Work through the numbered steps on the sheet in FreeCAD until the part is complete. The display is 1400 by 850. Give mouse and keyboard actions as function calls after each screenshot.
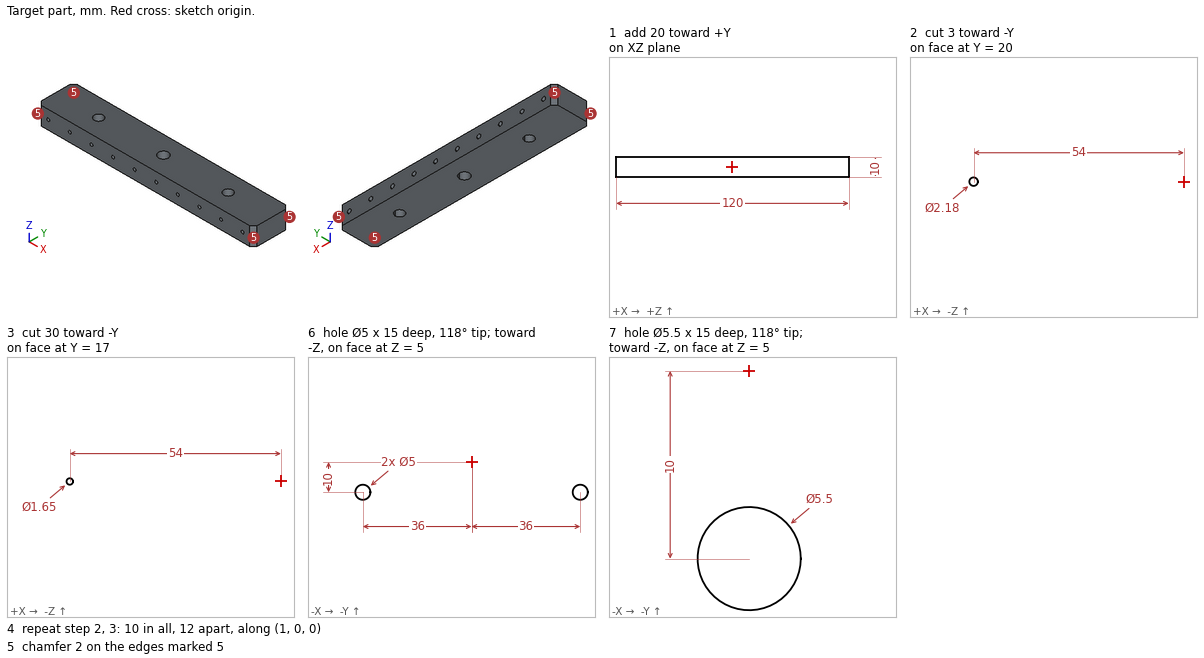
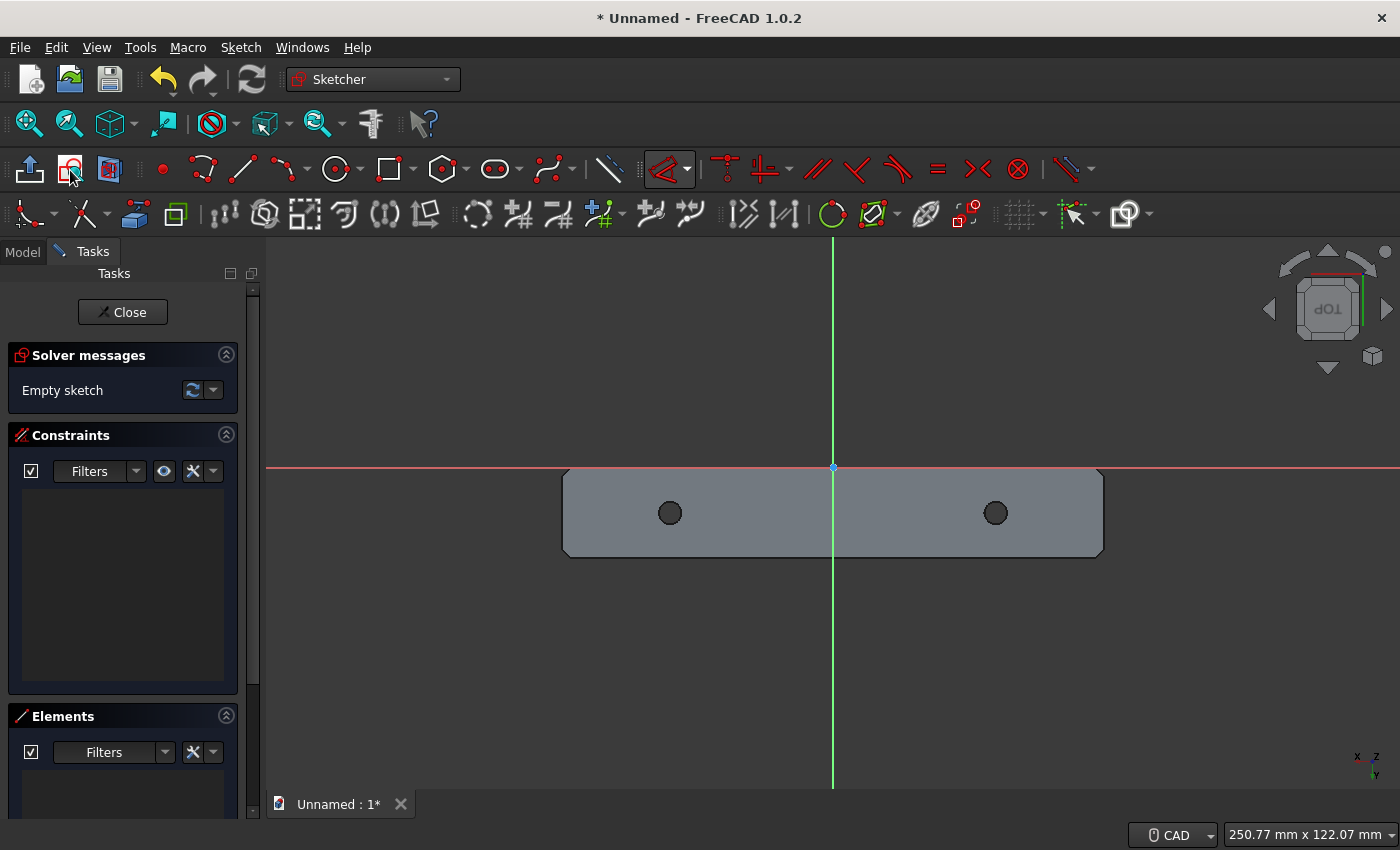
scroll(847, 493, up, 9)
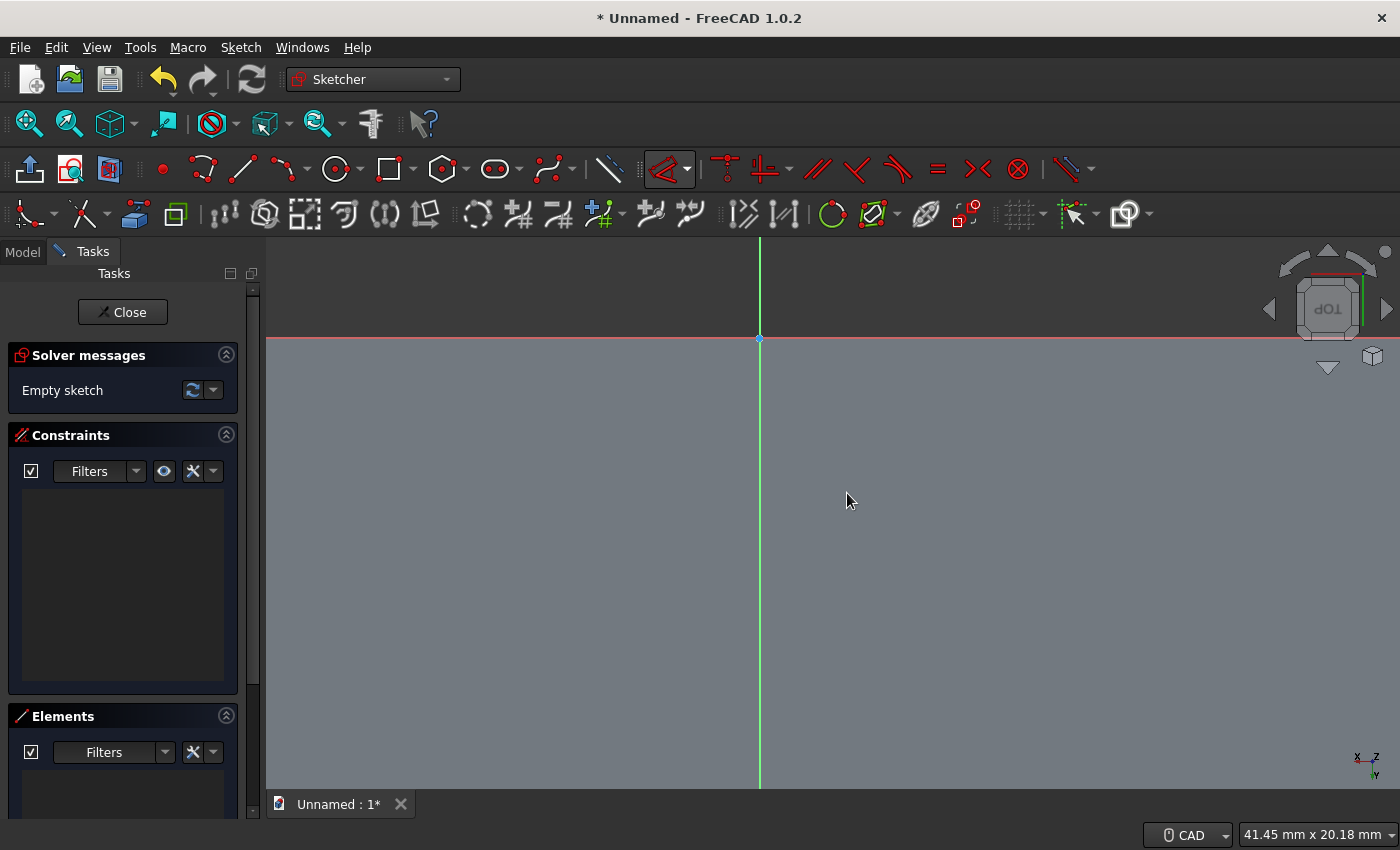
click(336, 170)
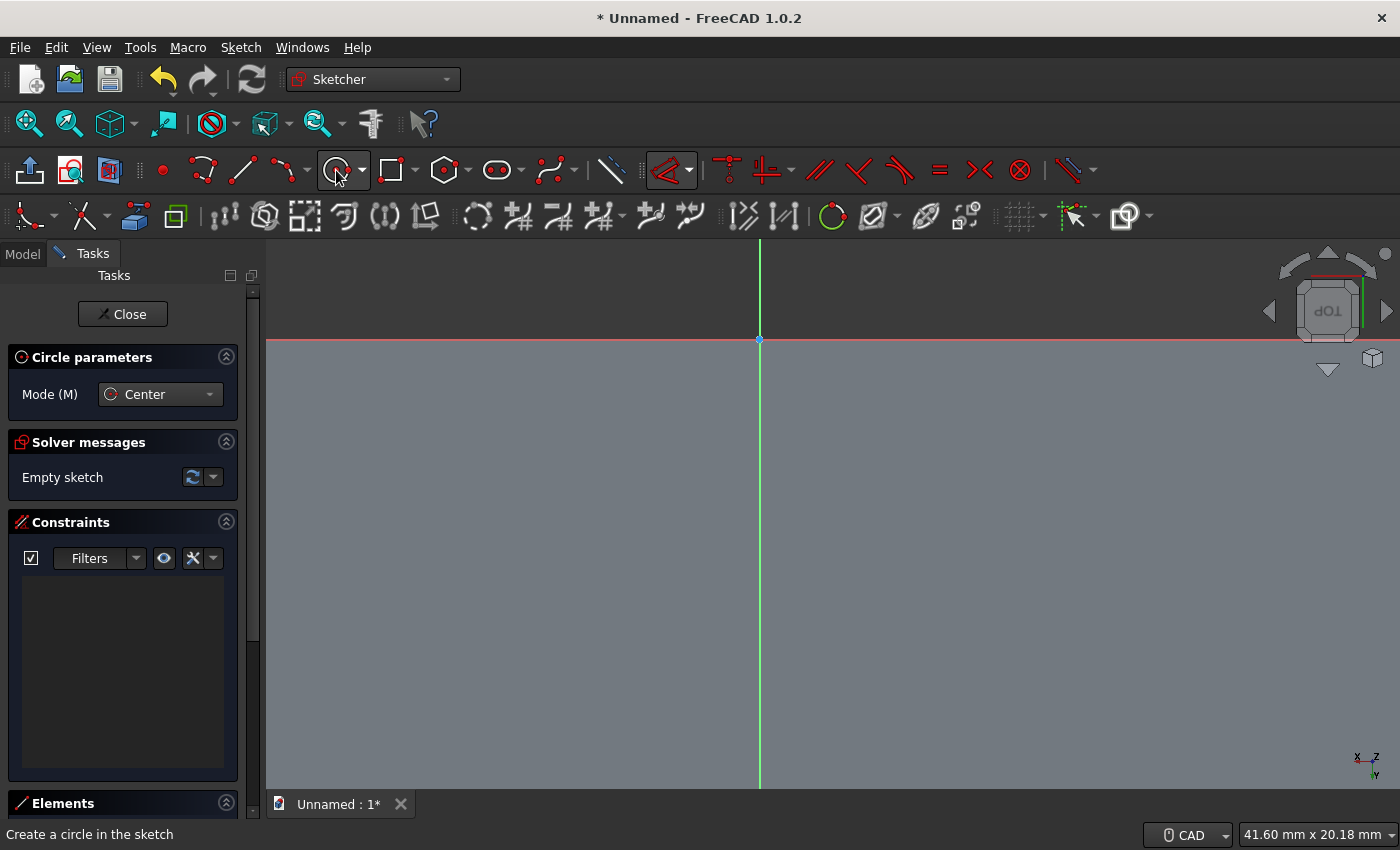
click(760, 612)
click(813, 559)
key(Escape)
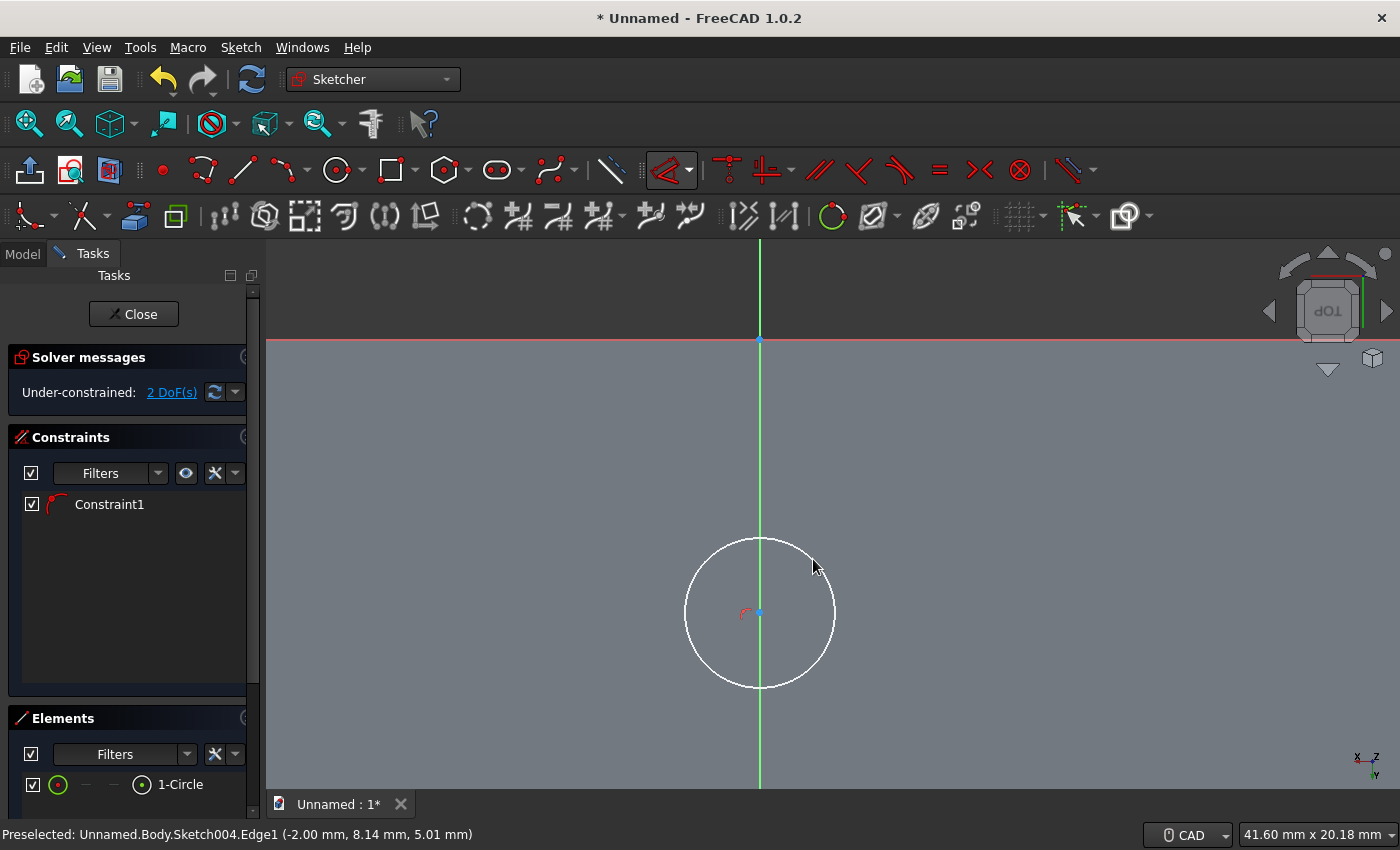
click(813, 560)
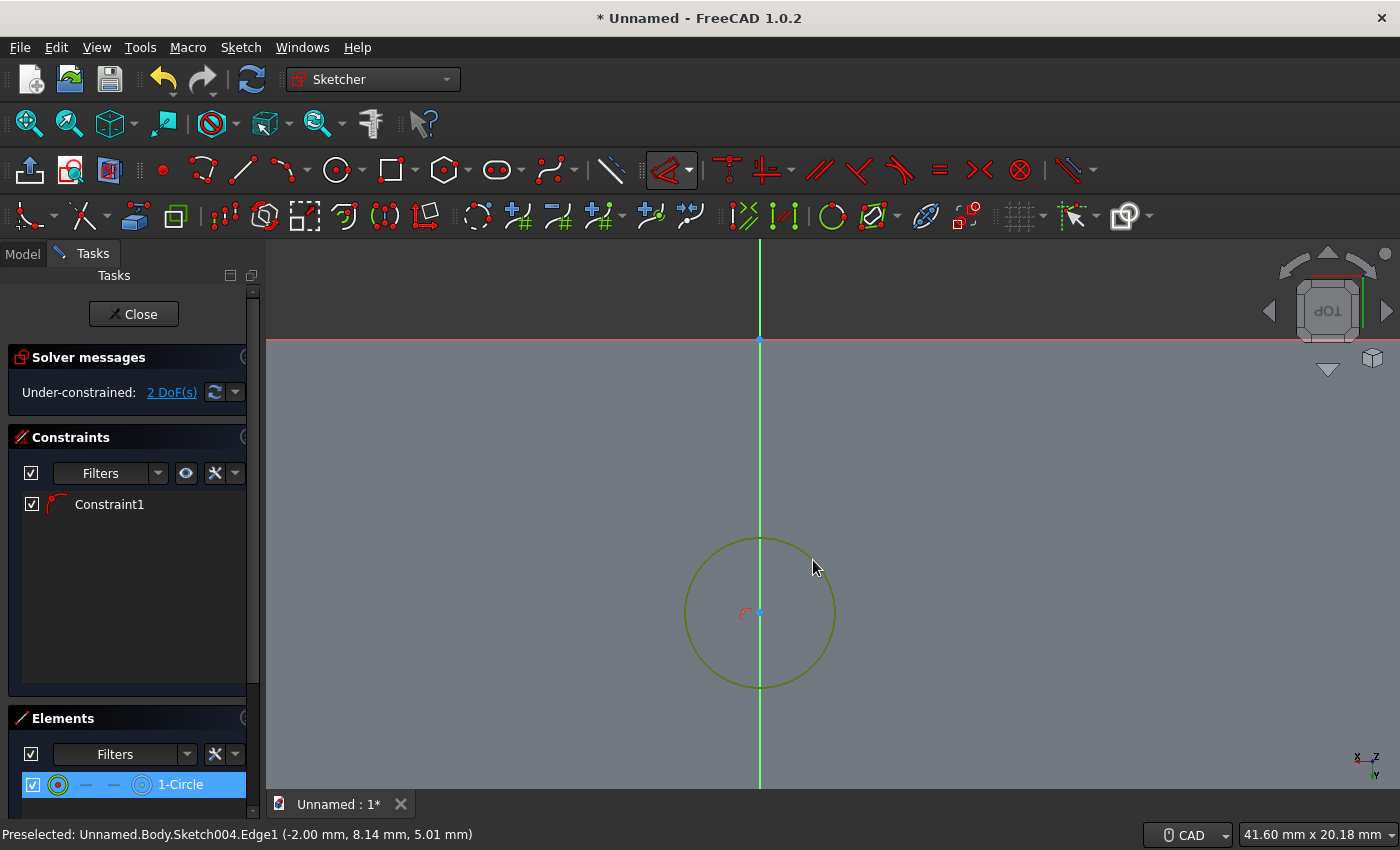
key(k)
key(o)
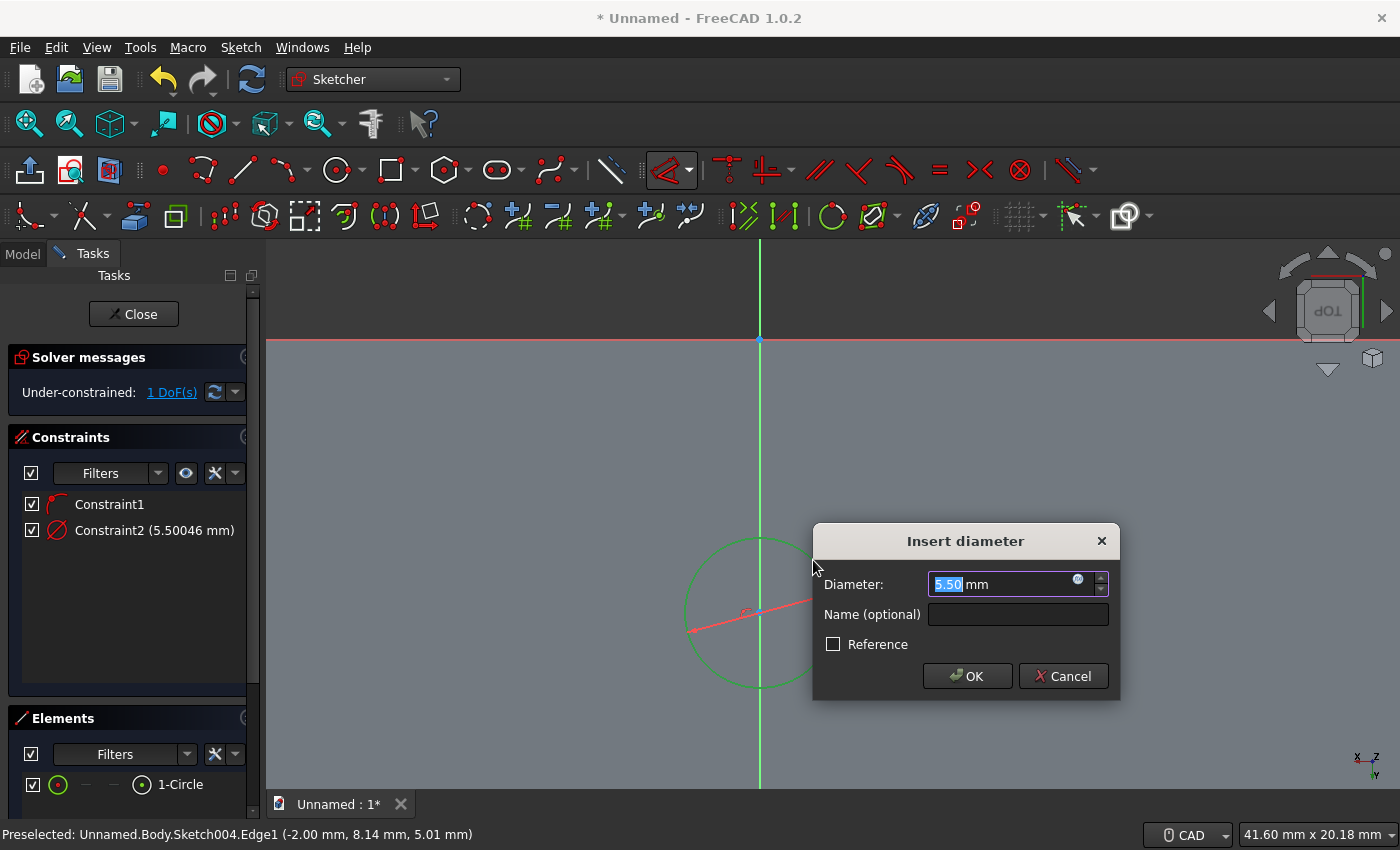
text(5.5)
key(Return)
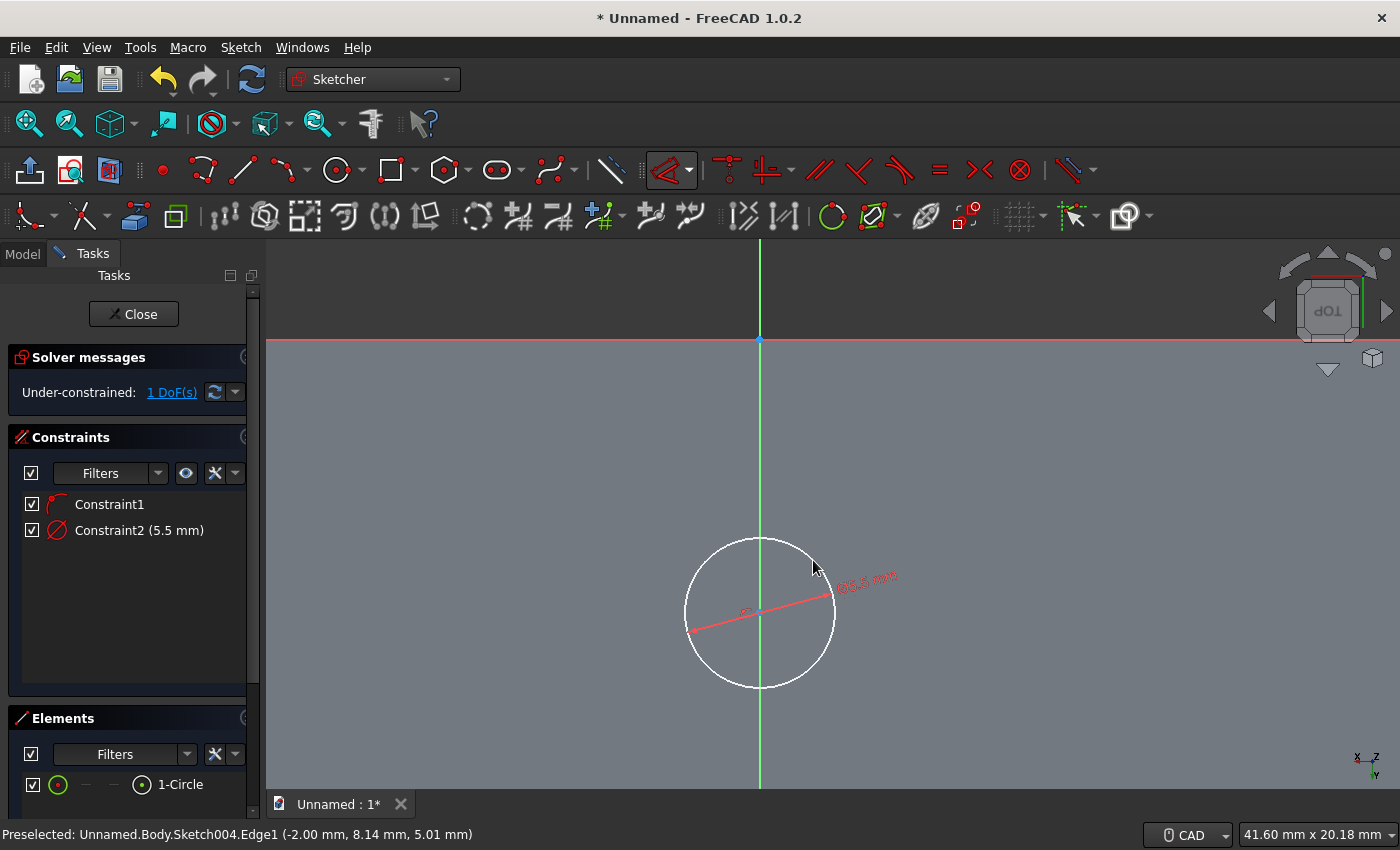
click(760, 613)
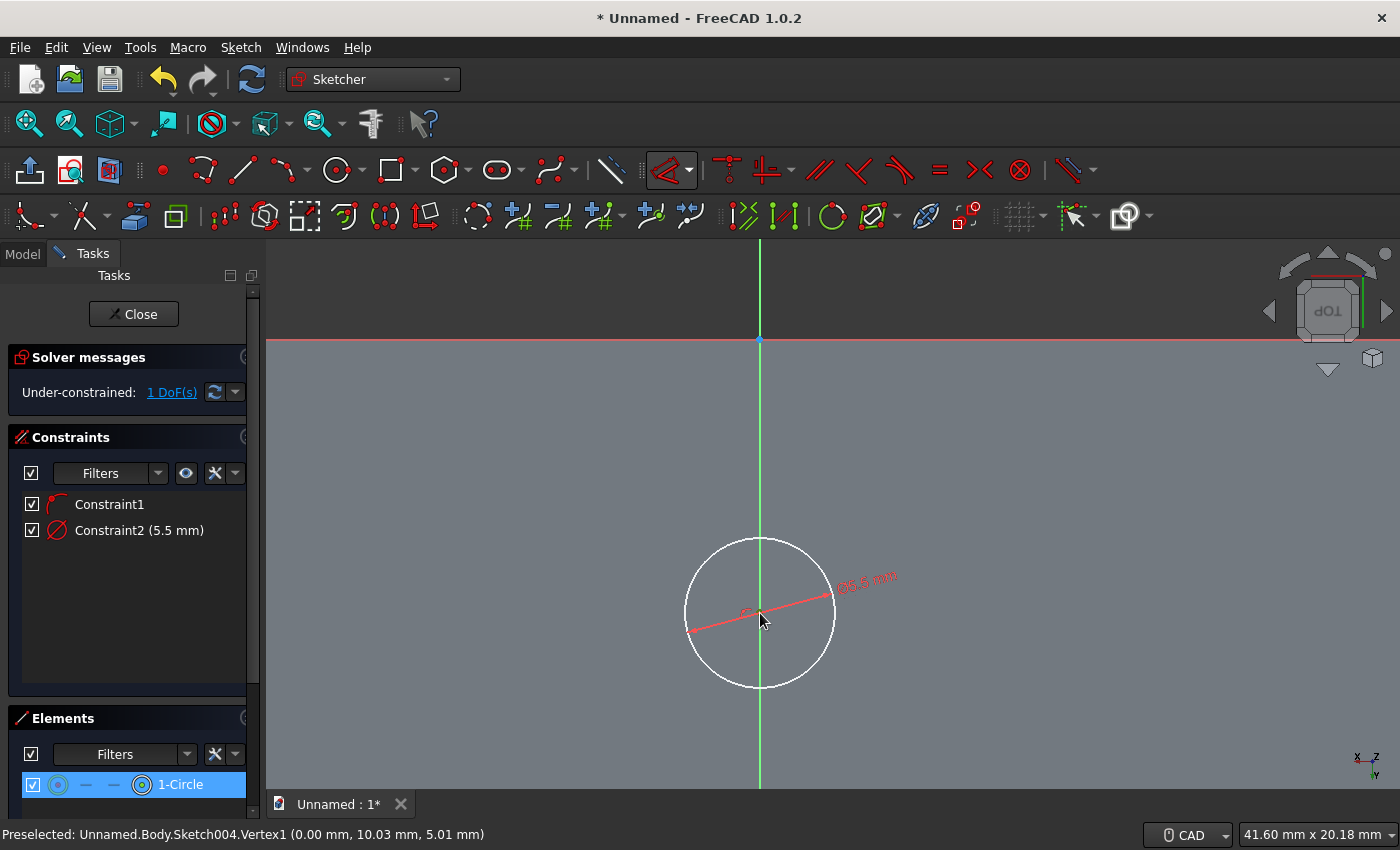
click(692, 170)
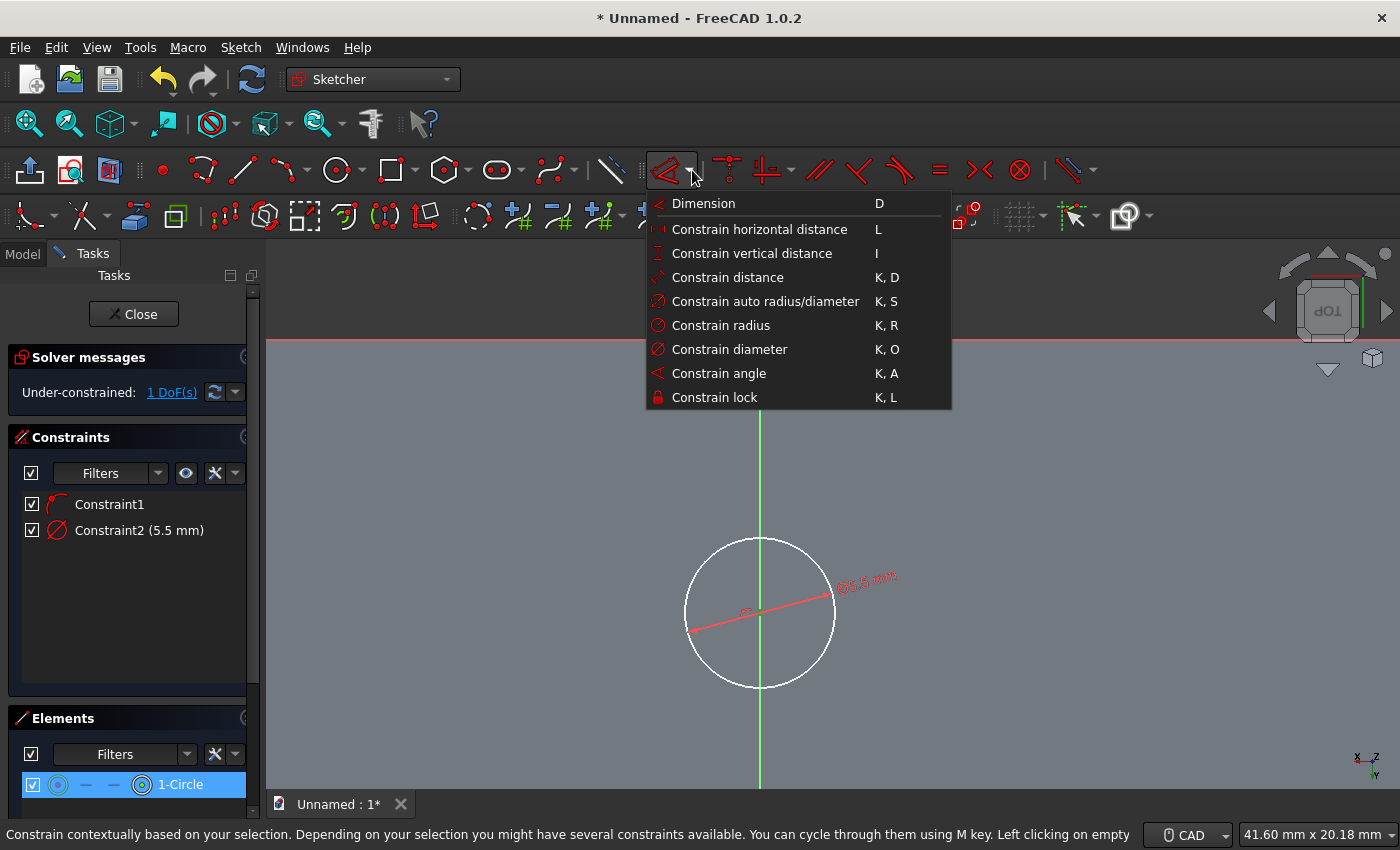
click(799, 253)